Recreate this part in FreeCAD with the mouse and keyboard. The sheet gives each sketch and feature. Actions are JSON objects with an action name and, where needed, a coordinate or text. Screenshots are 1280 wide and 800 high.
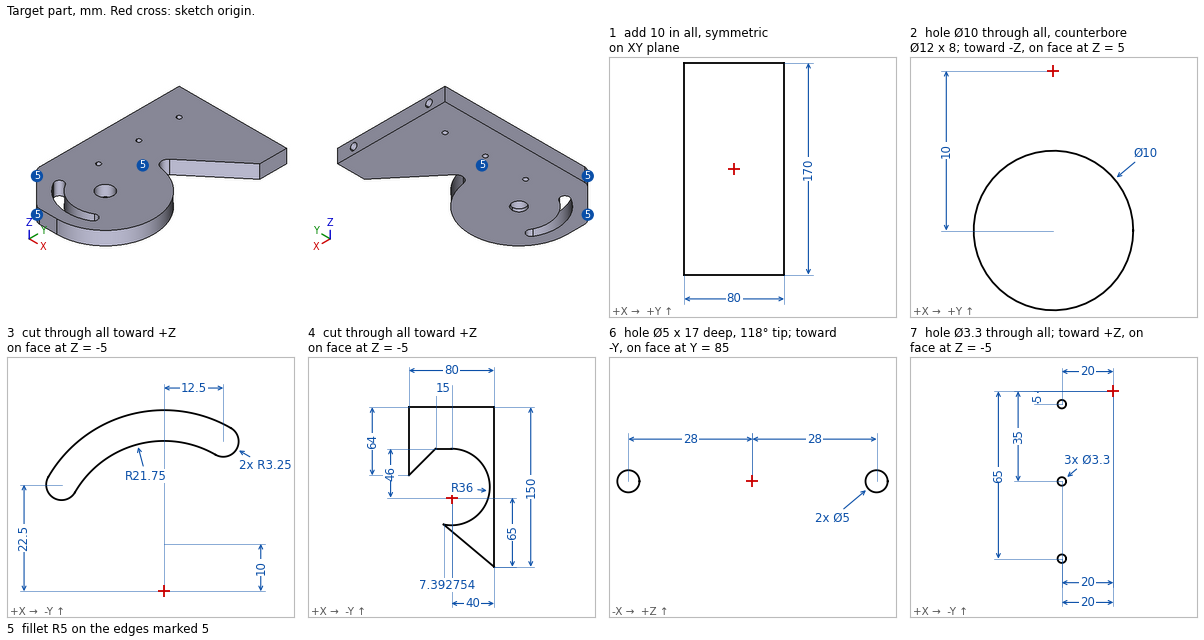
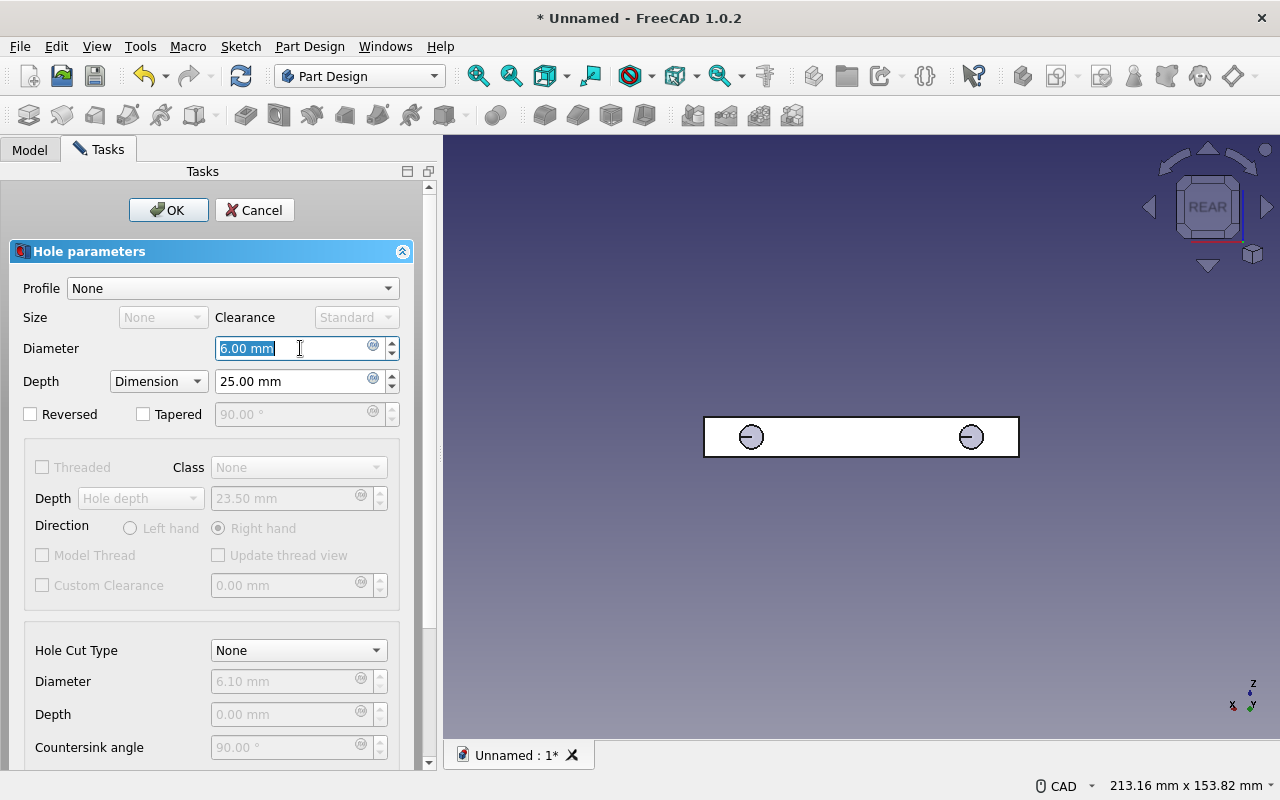
{"action": "type", "text": "5"}
{"action": "key", "text": "Tab"}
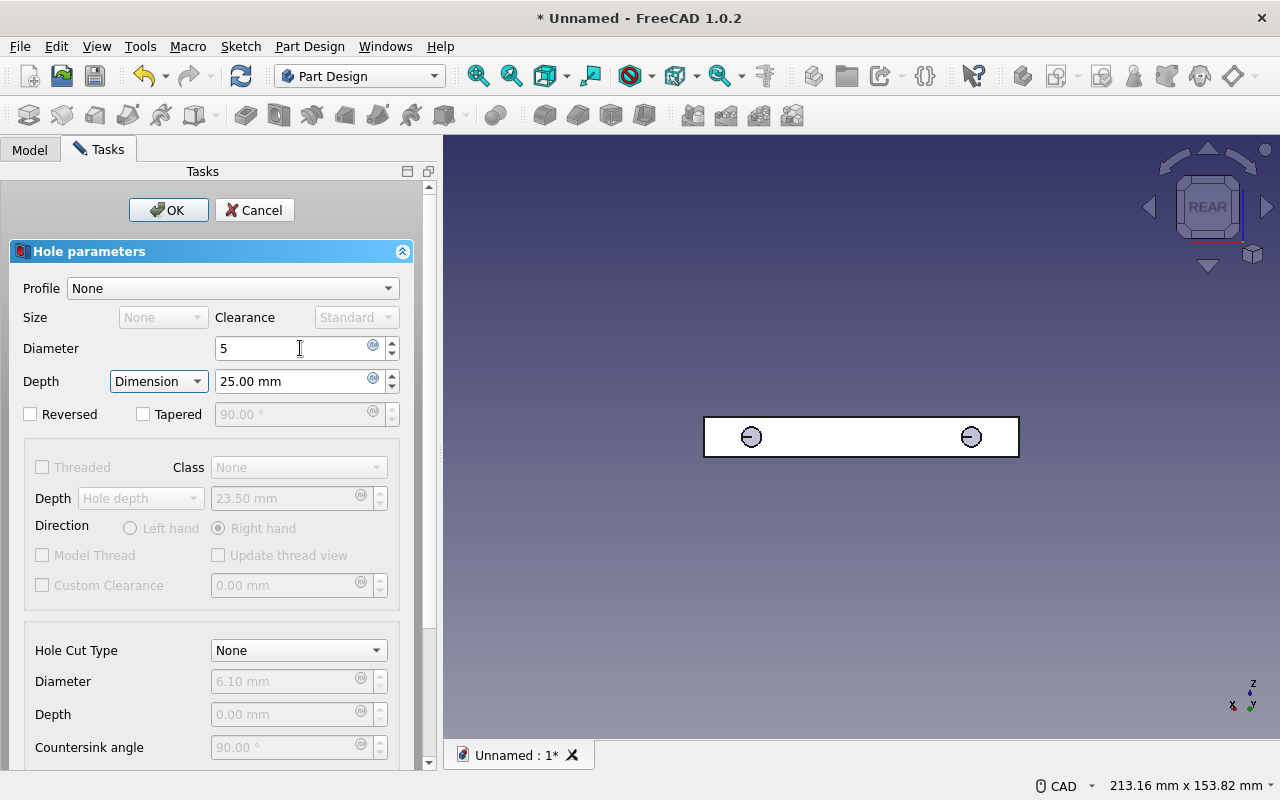
{"action": "triple_click", "coordinate": [300, 382]}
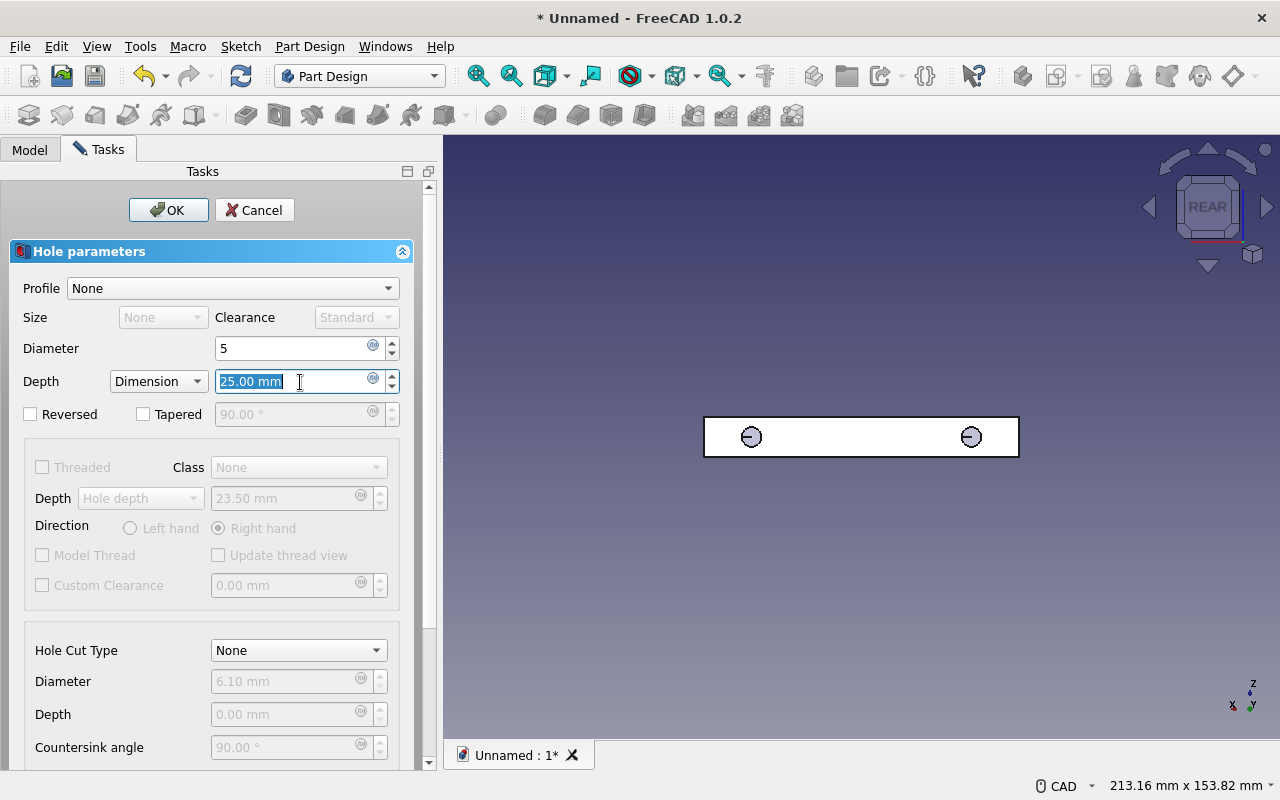
{"action": "type", "text": "17"}
{"action": "key", "text": "Tab"}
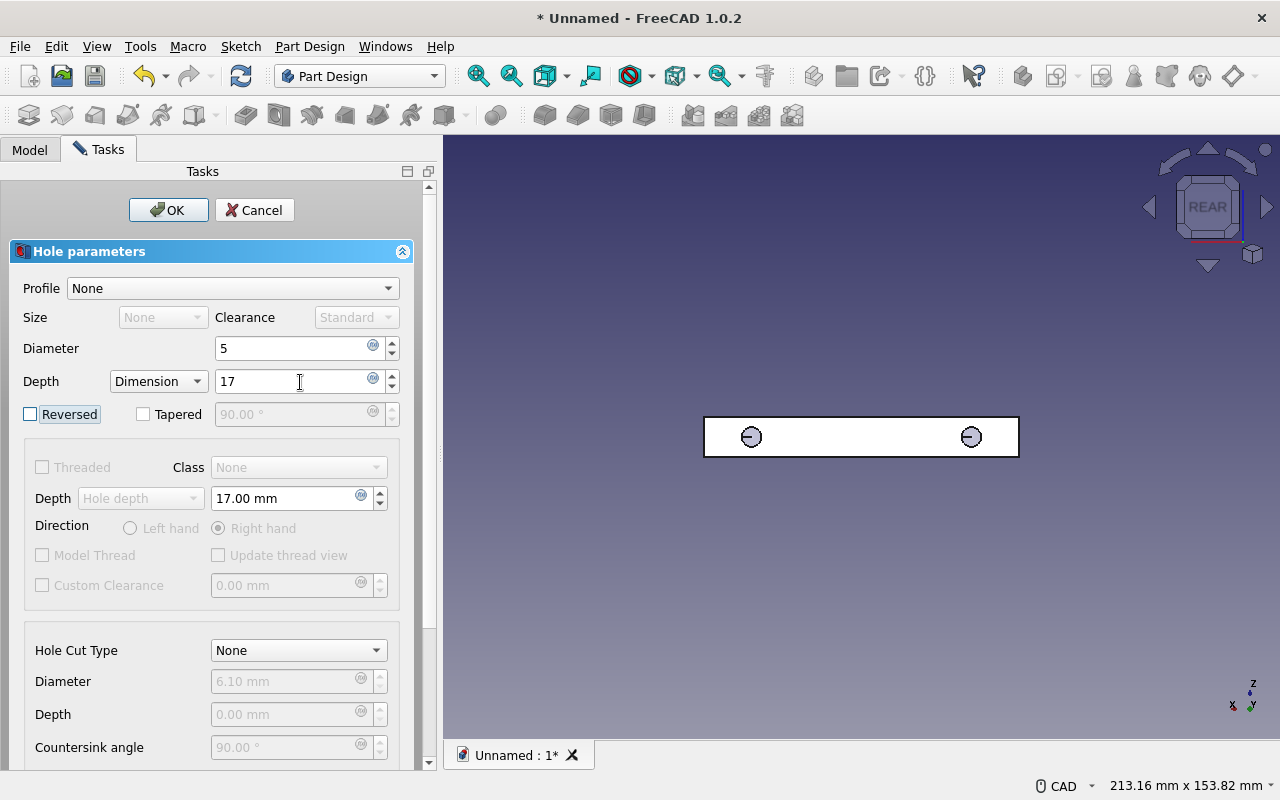
{"action": "left_click", "coordinate": [169, 210]}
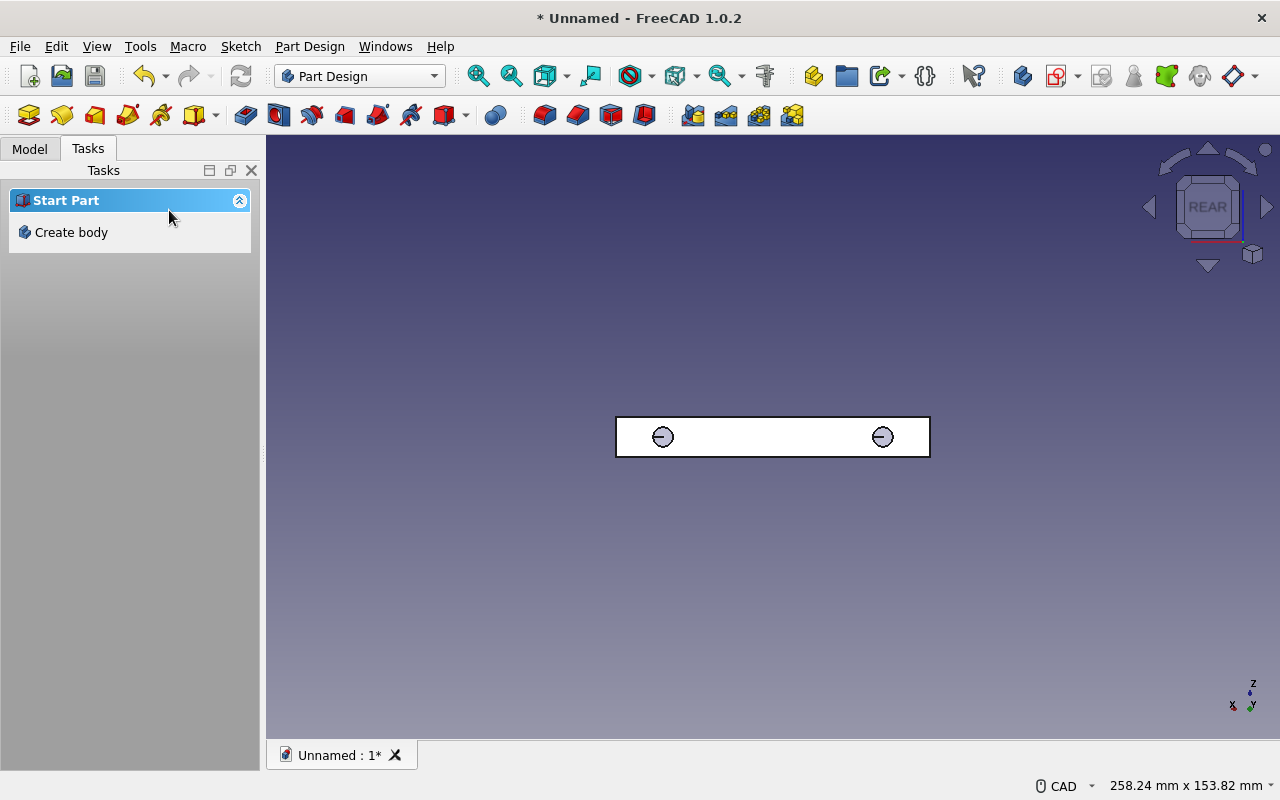
{"action": "left_click", "coordinate": [479, 76]}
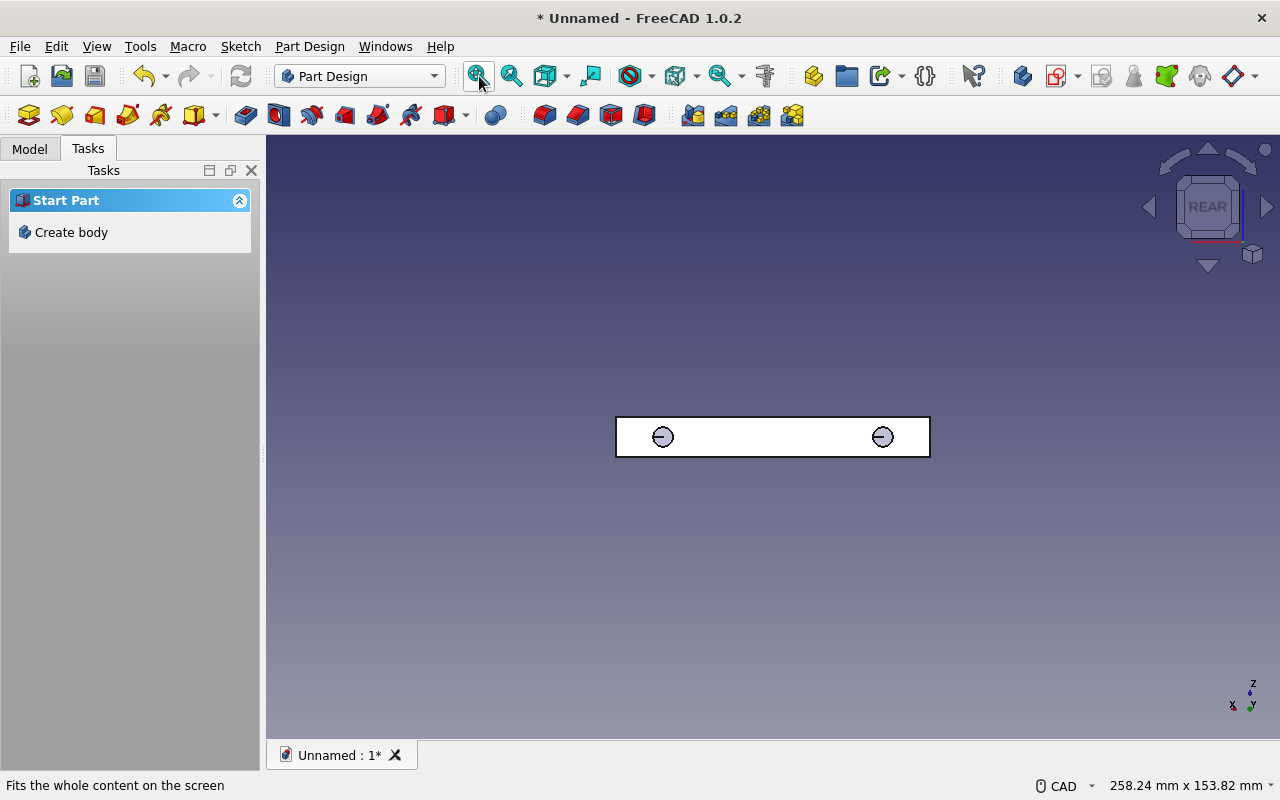
{"action": "key", "text": "5"}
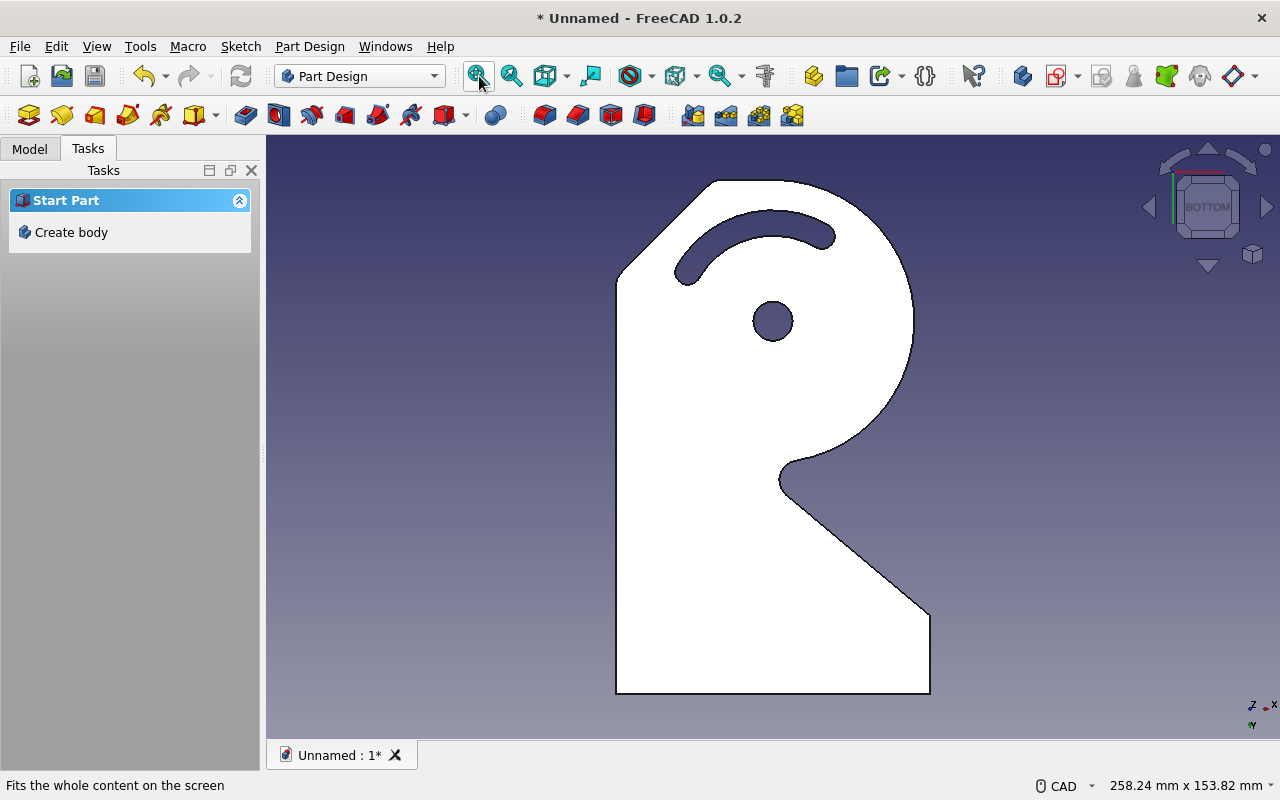
{"action": "left_click", "coordinate": [728, 583]}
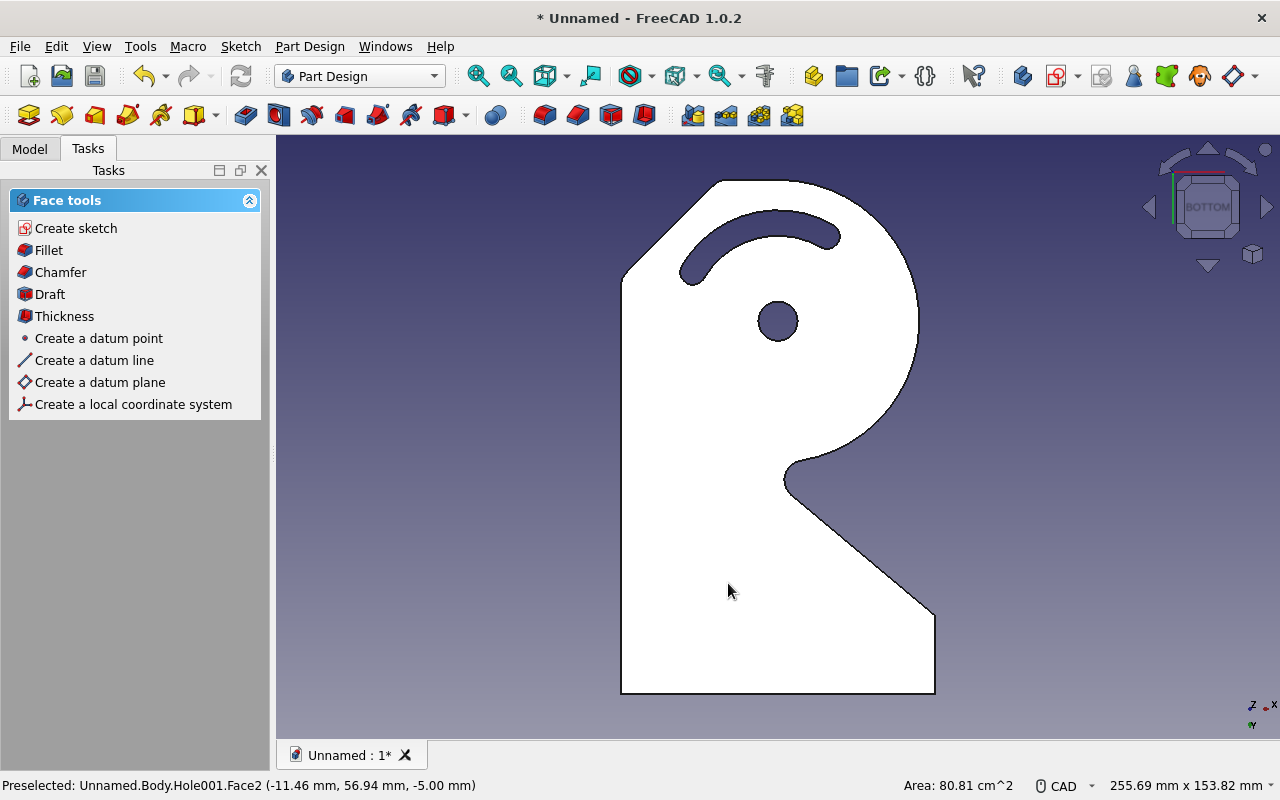
{"action": "left_click", "coordinate": [1056, 76]}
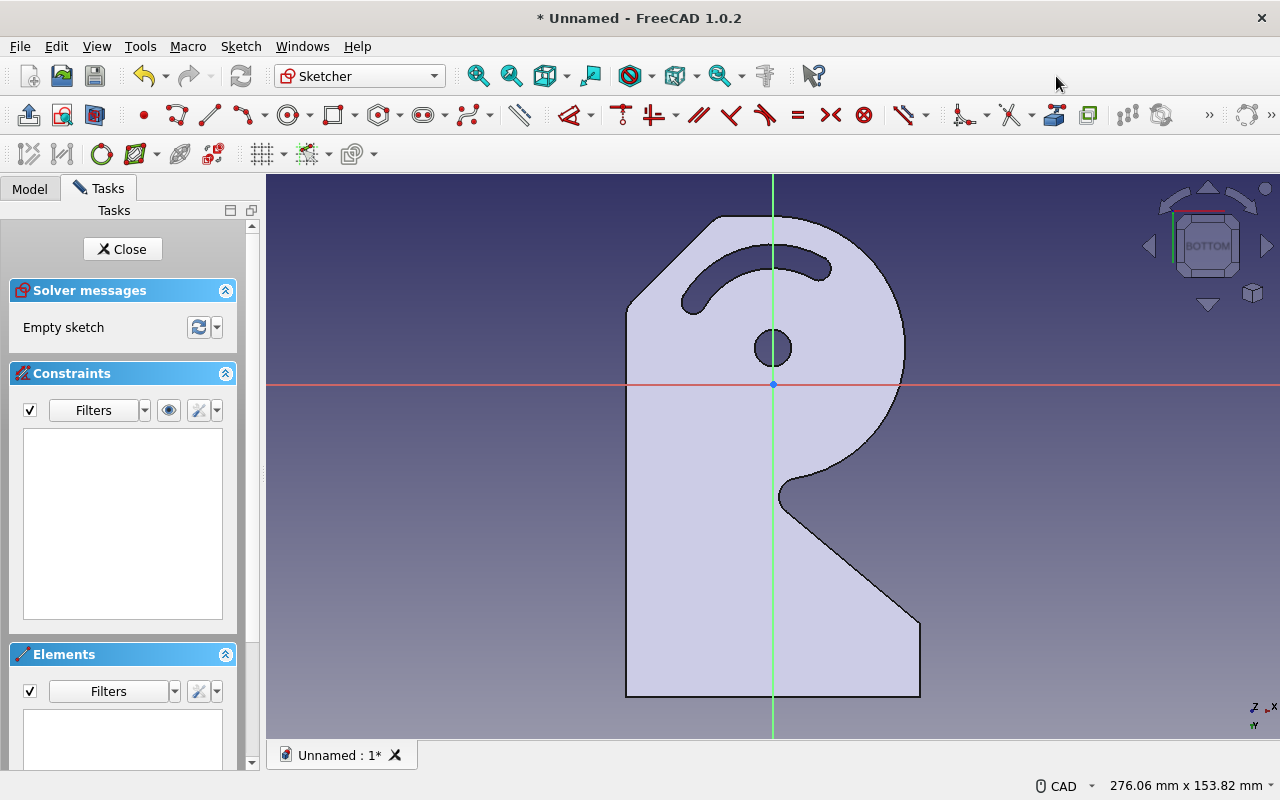
{"action": "scroll", "coordinate": [792, 611], "scroll_direction": "up", "scroll_amount": 2}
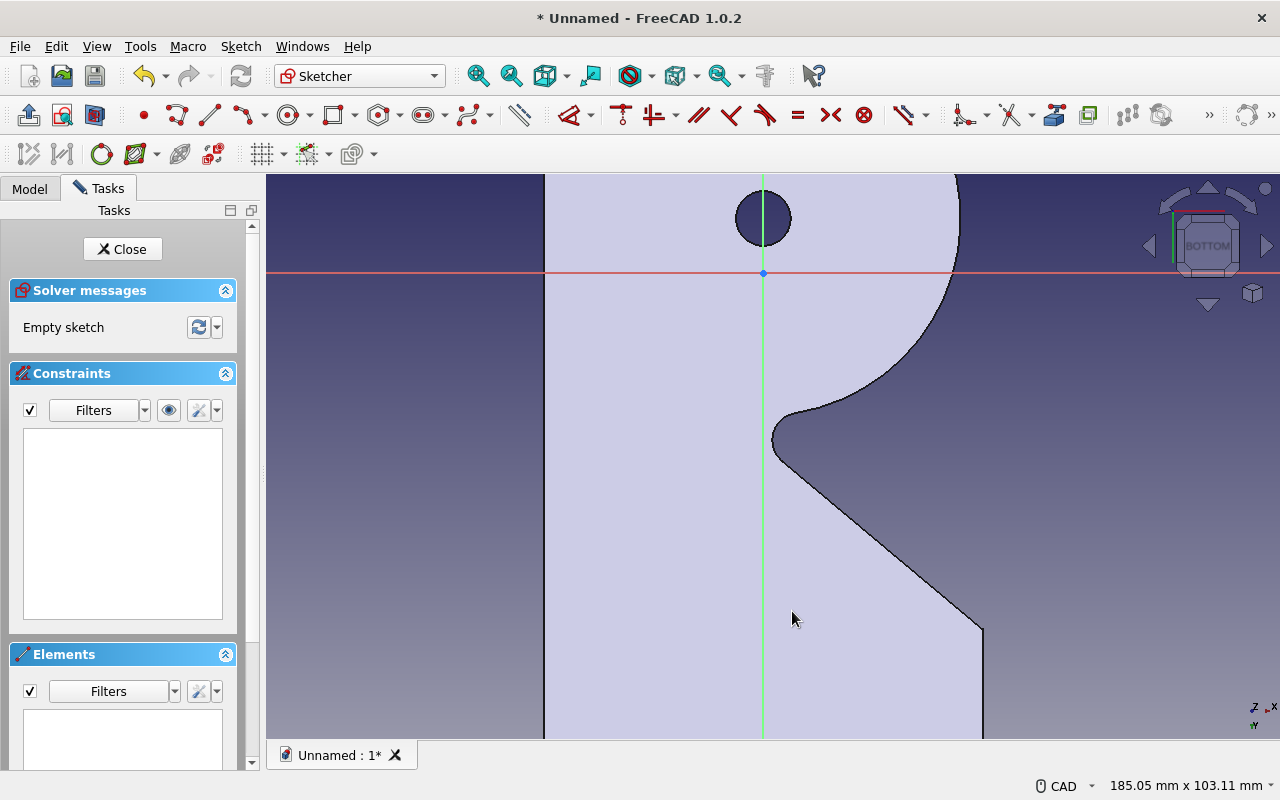
{"action": "left_click", "coordinate": [288, 116]}